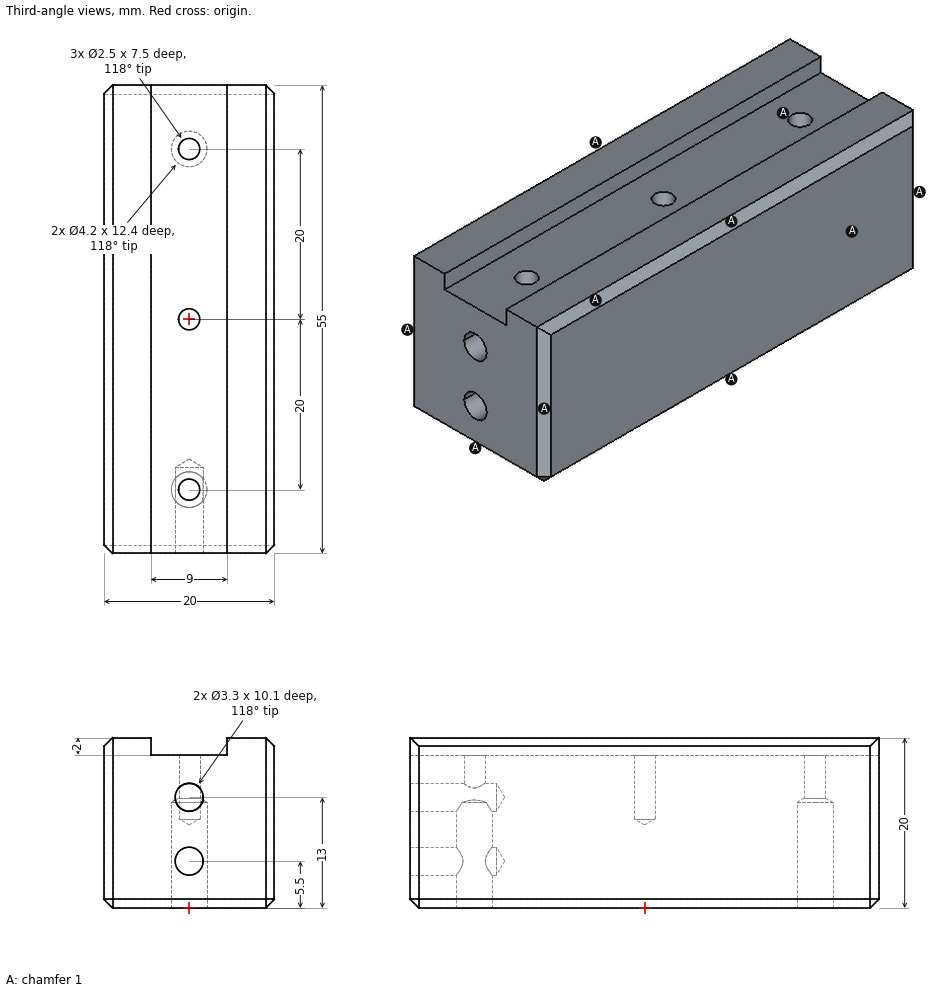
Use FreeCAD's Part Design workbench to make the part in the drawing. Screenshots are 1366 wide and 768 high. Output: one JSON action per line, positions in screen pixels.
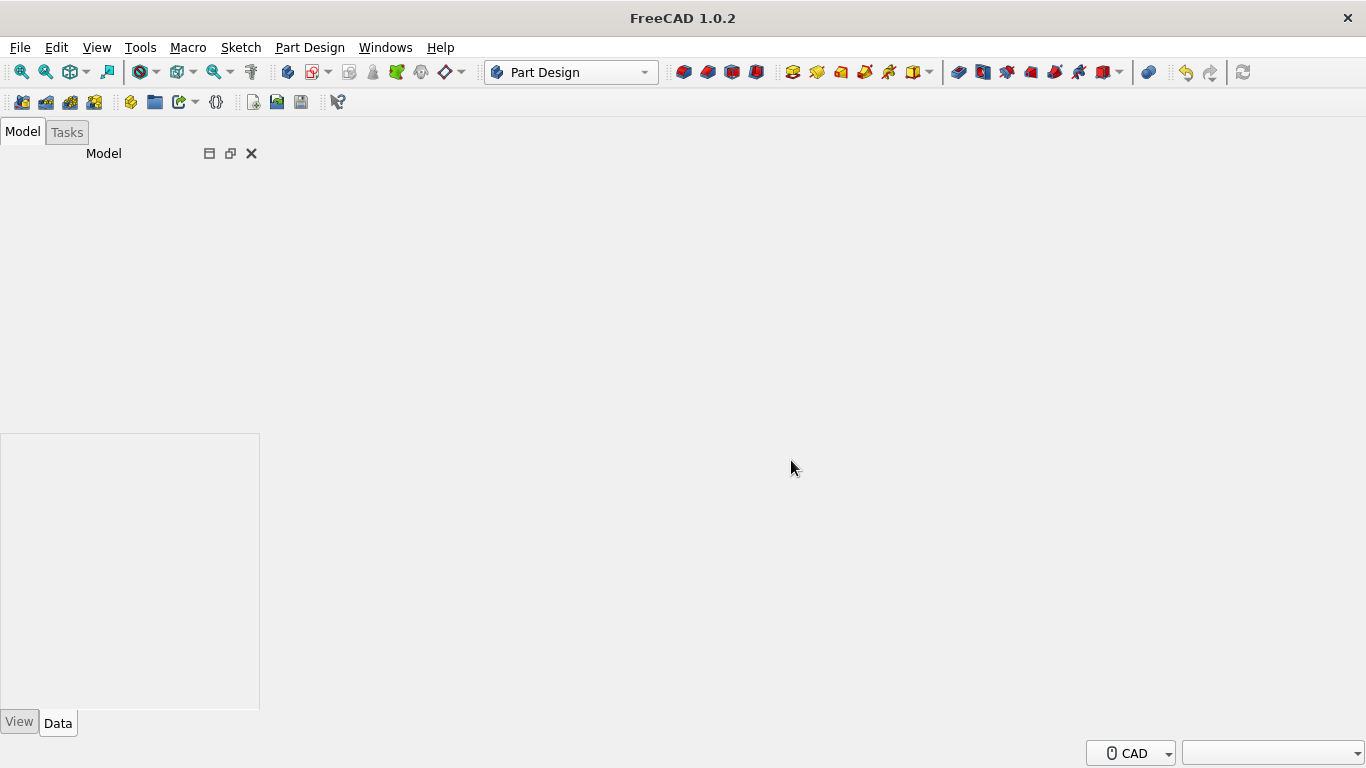
{"action": "left_click", "coordinate": [254, 102]}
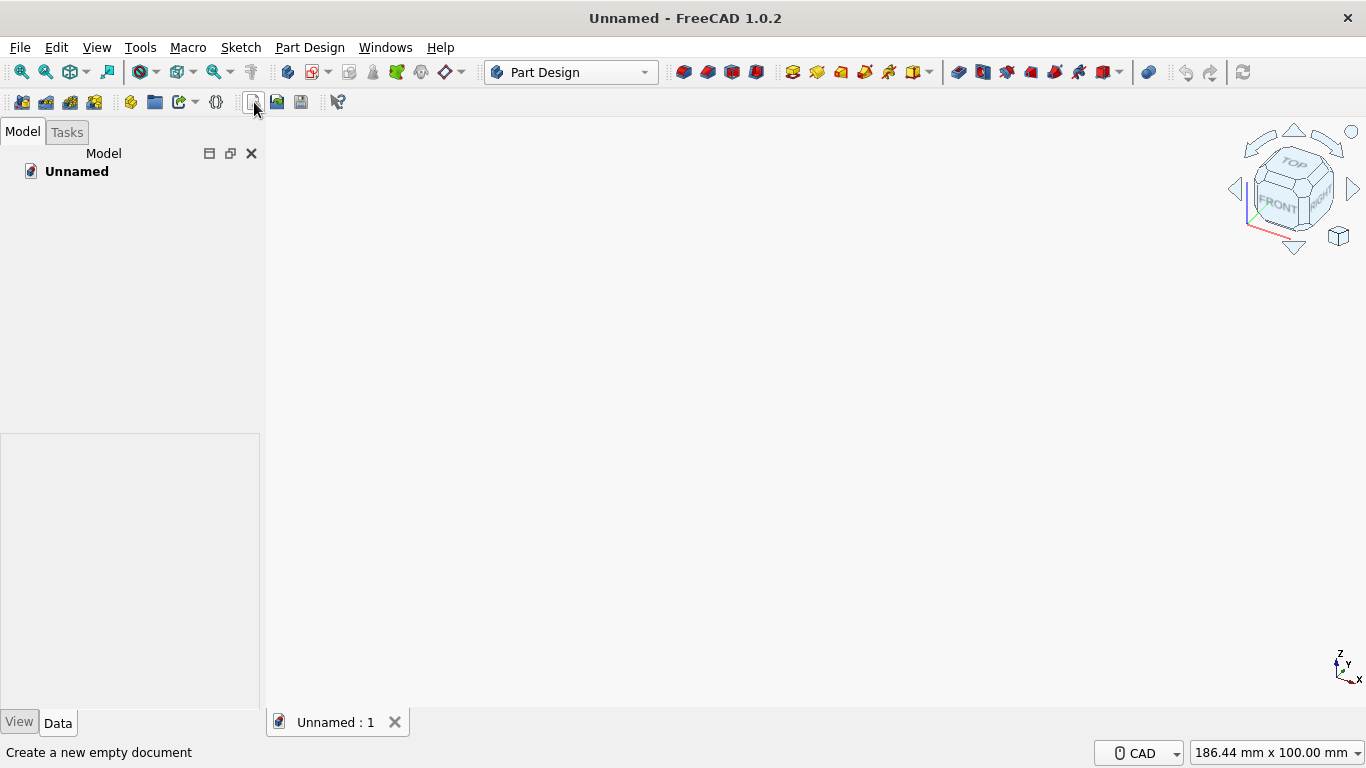
{"action": "left_click", "coordinate": [312, 72]}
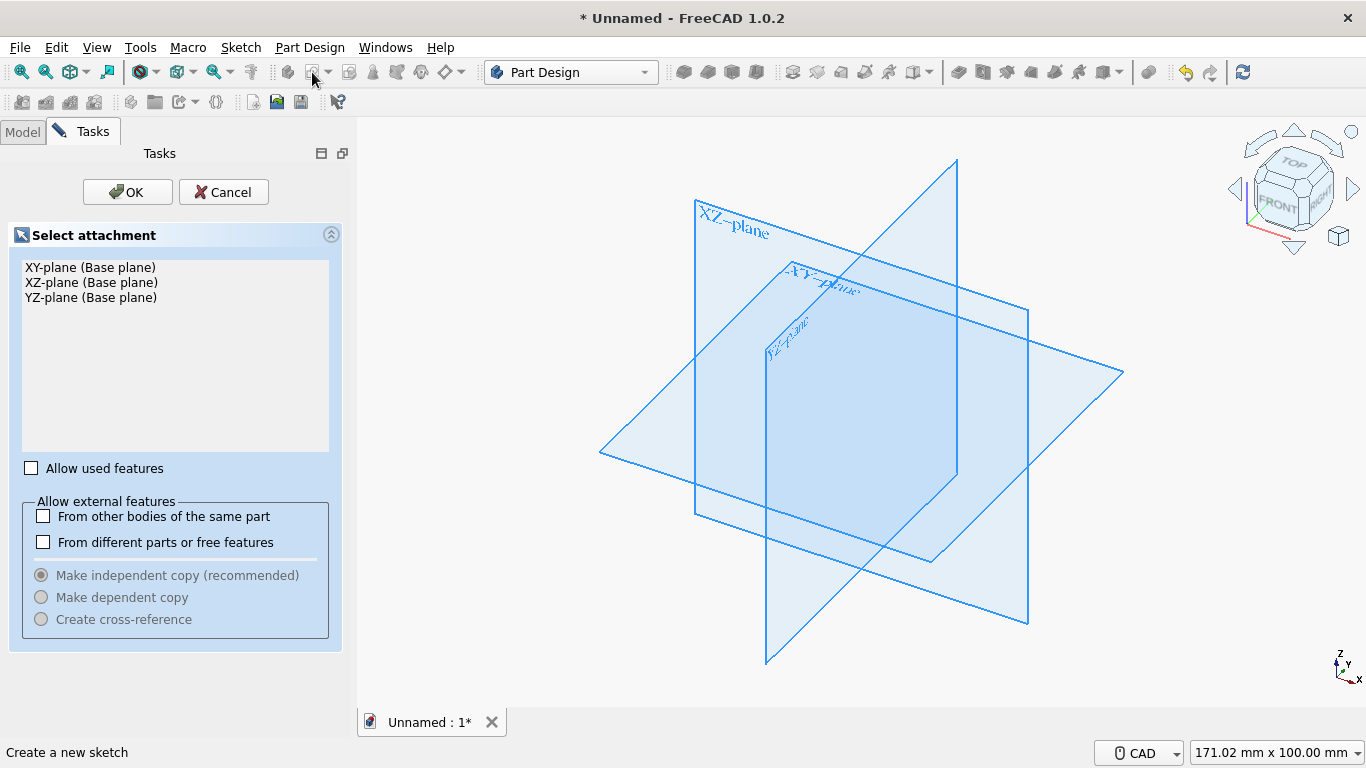
{"action": "left_click", "coordinate": [82, 268]}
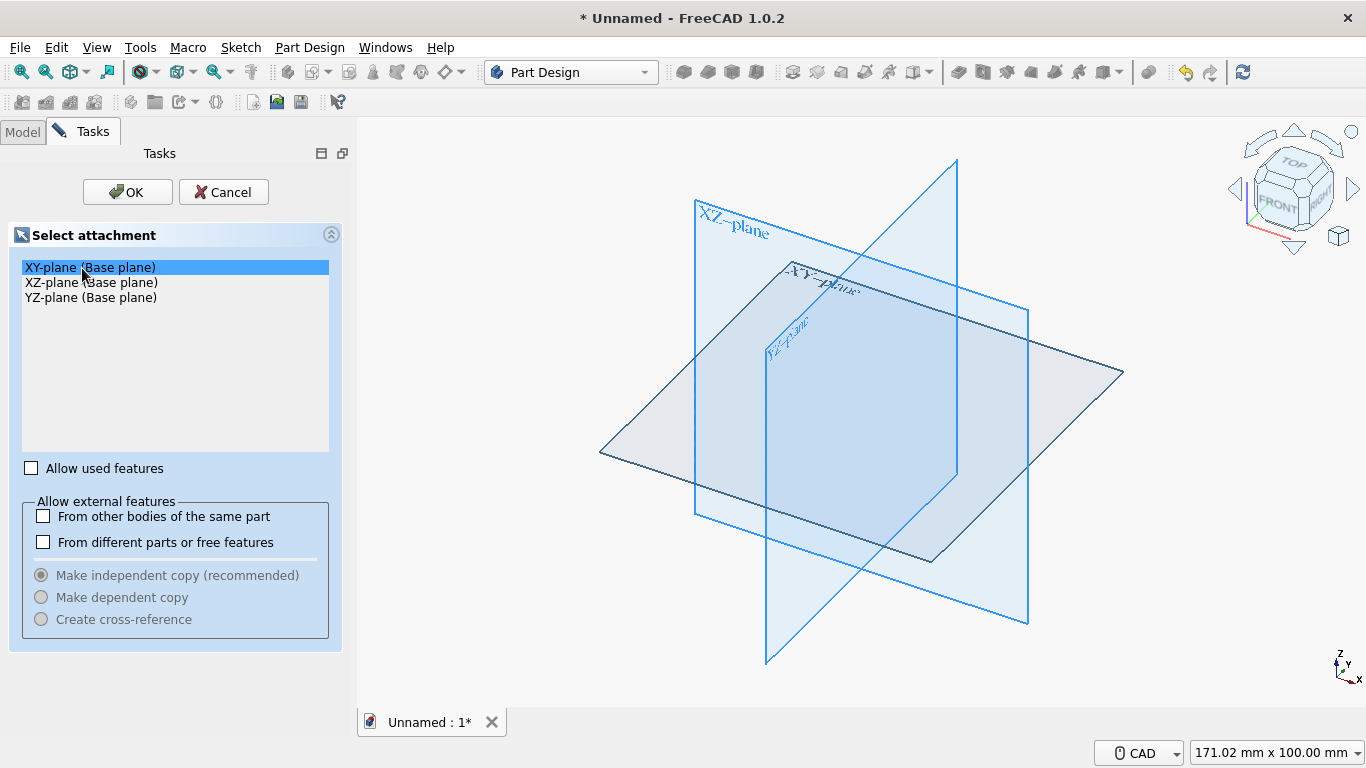
{"action": "left_click", "coordinate": [128, 192]}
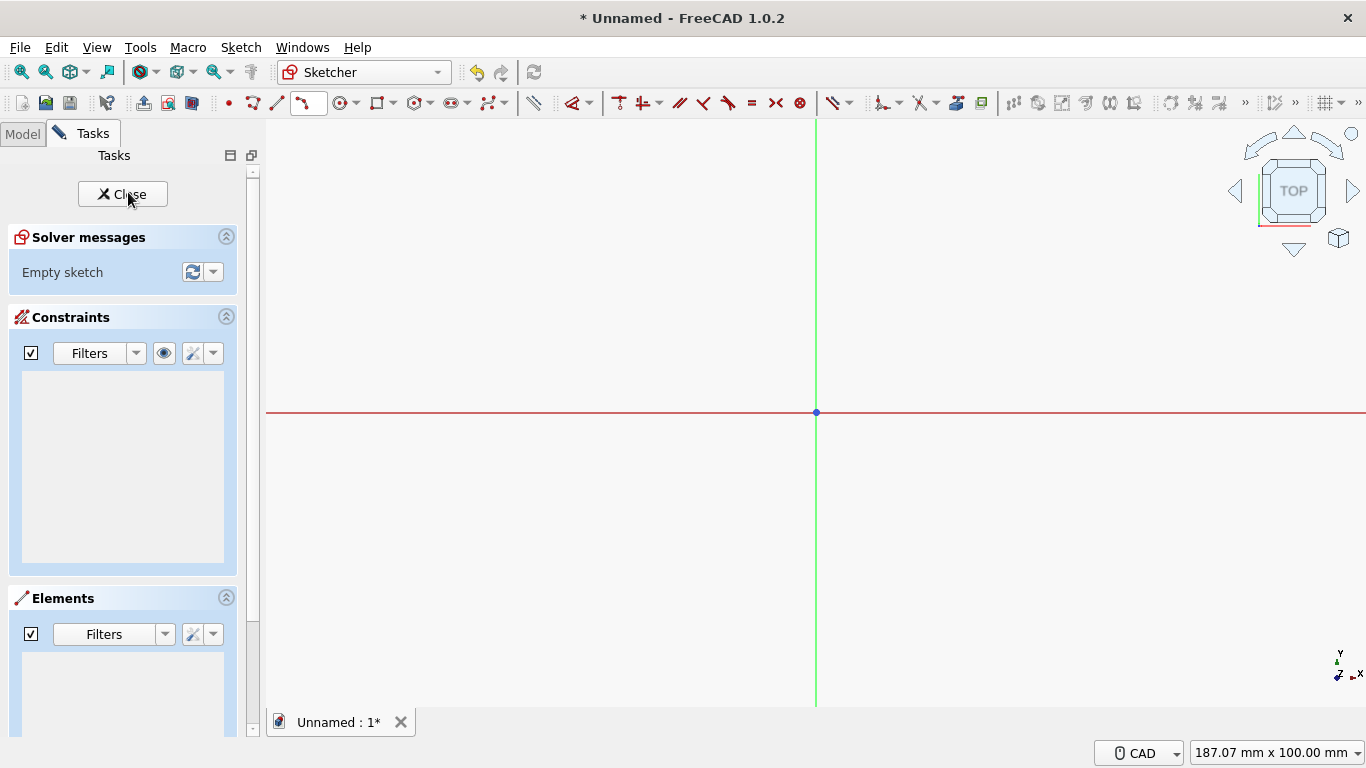
{"action": "key", "text": "g v"}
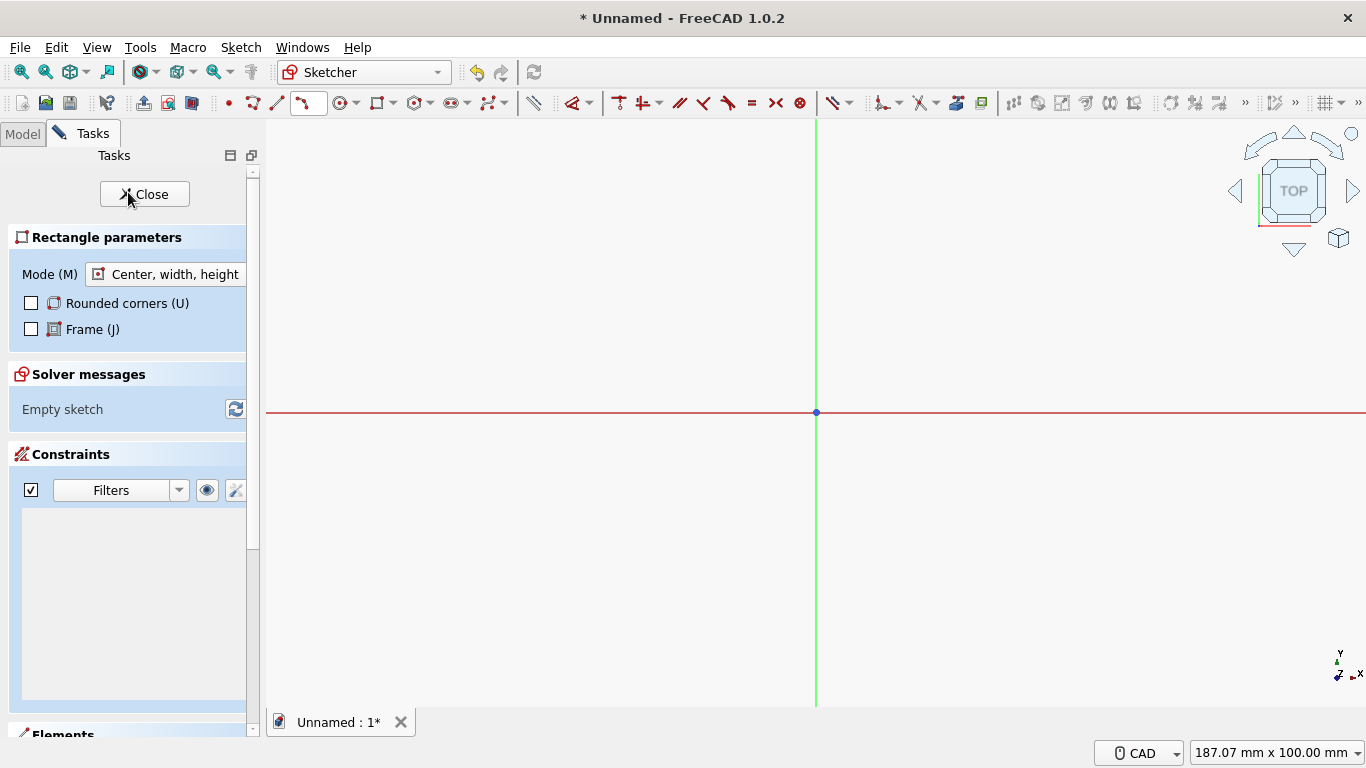
{"action": "left_click", "coordinate": [816, 413]}
{"action": "mouse_move", "coordinate": [875, 251]}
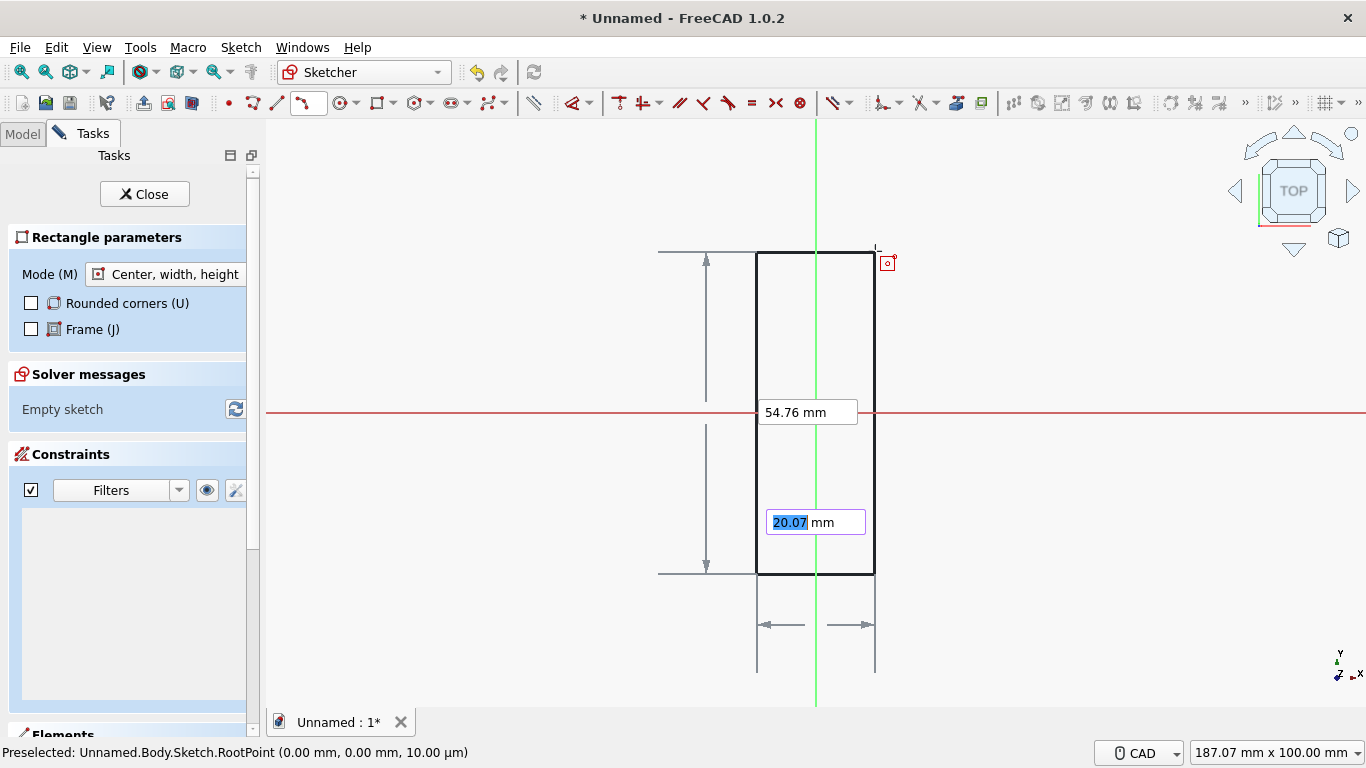
{"action": "type", "text": "20"}
{"action": "key", "text": "Tab"}
{"action": "type", "text": "55"}
{"action": "key", "text": "Return"}
{"action": "key", "text": "Escape"}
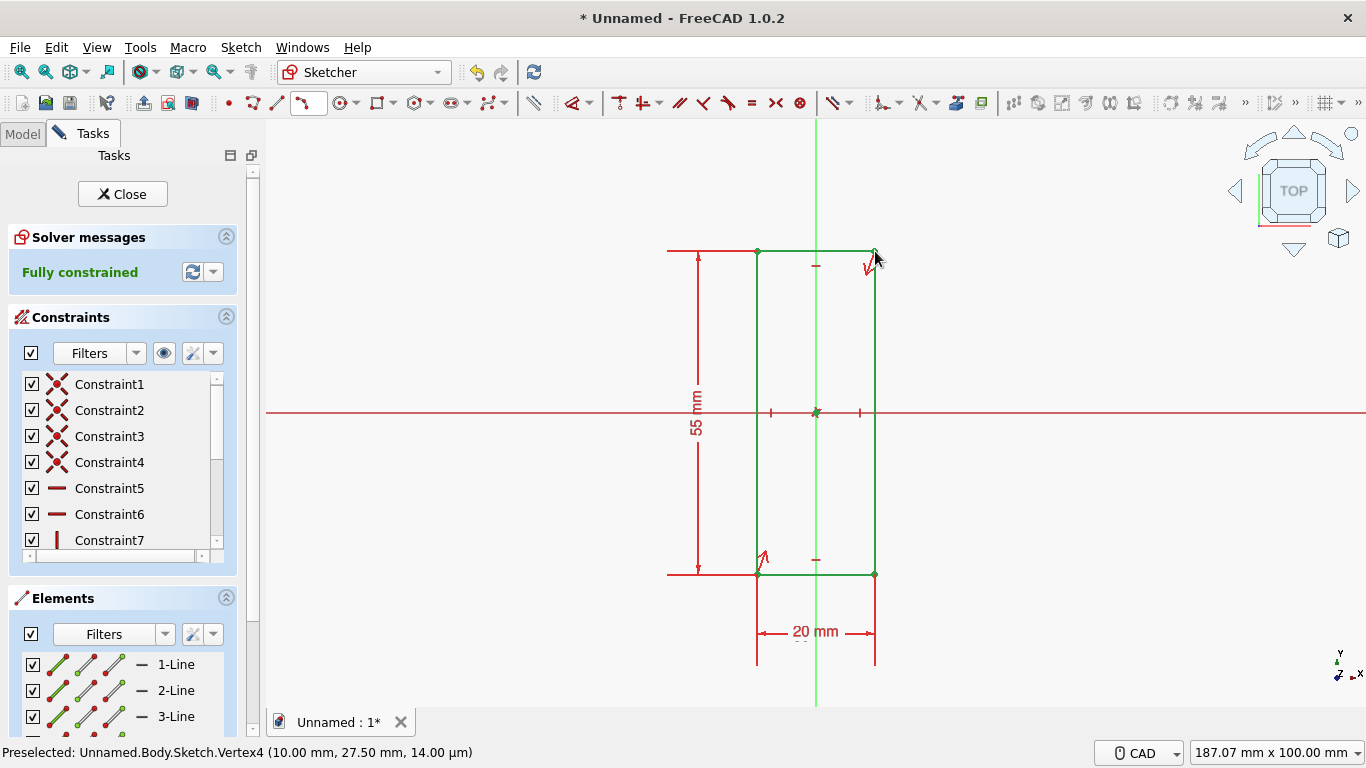
{"action": "left_click", "coordinate": [123, 194]}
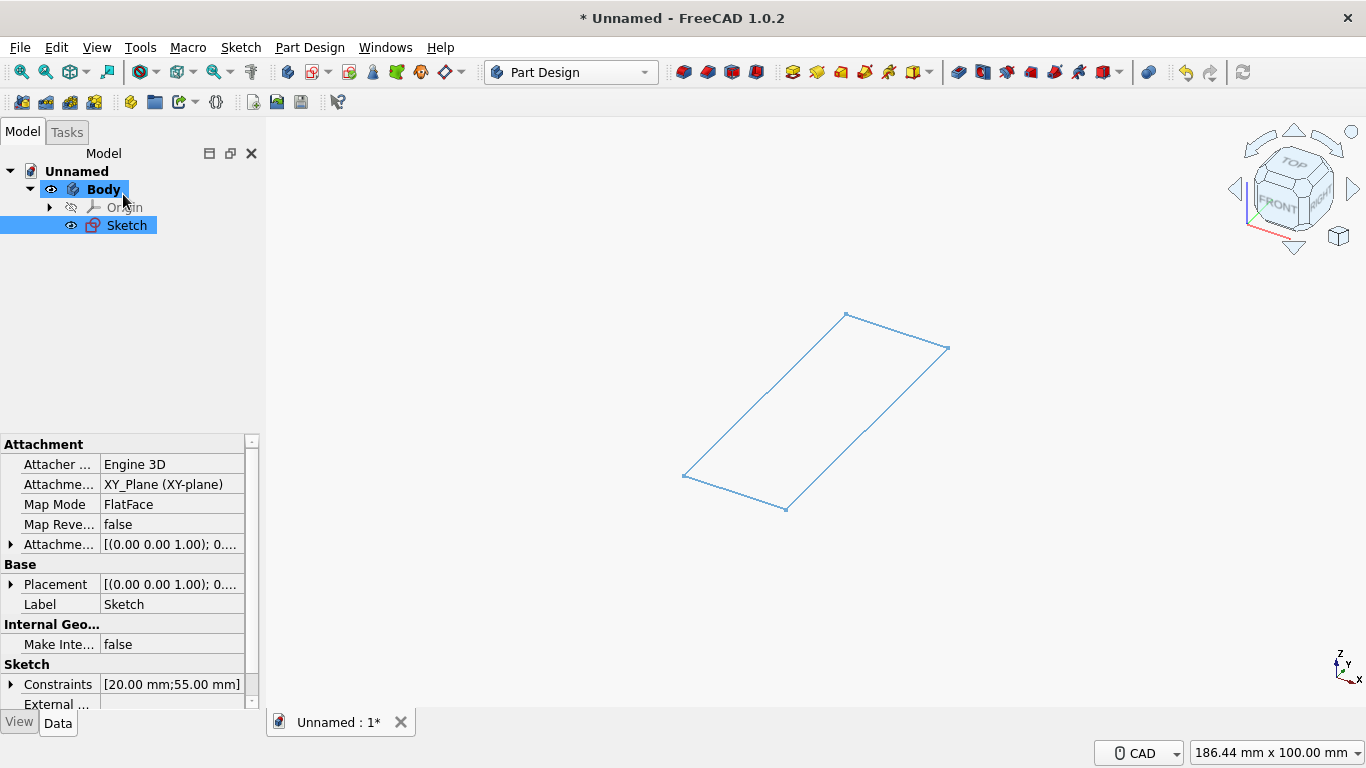
{"action": "left_click", "coordinate": [794, 72]}